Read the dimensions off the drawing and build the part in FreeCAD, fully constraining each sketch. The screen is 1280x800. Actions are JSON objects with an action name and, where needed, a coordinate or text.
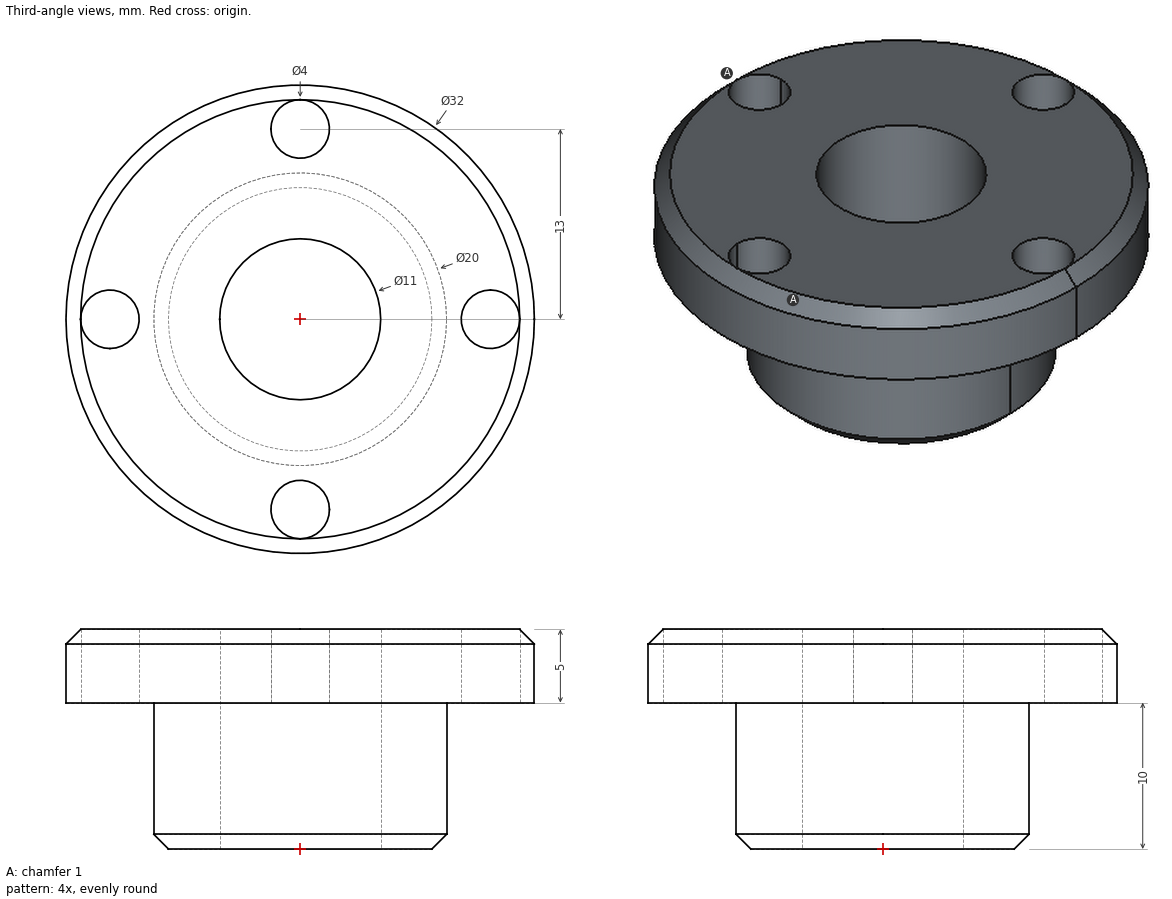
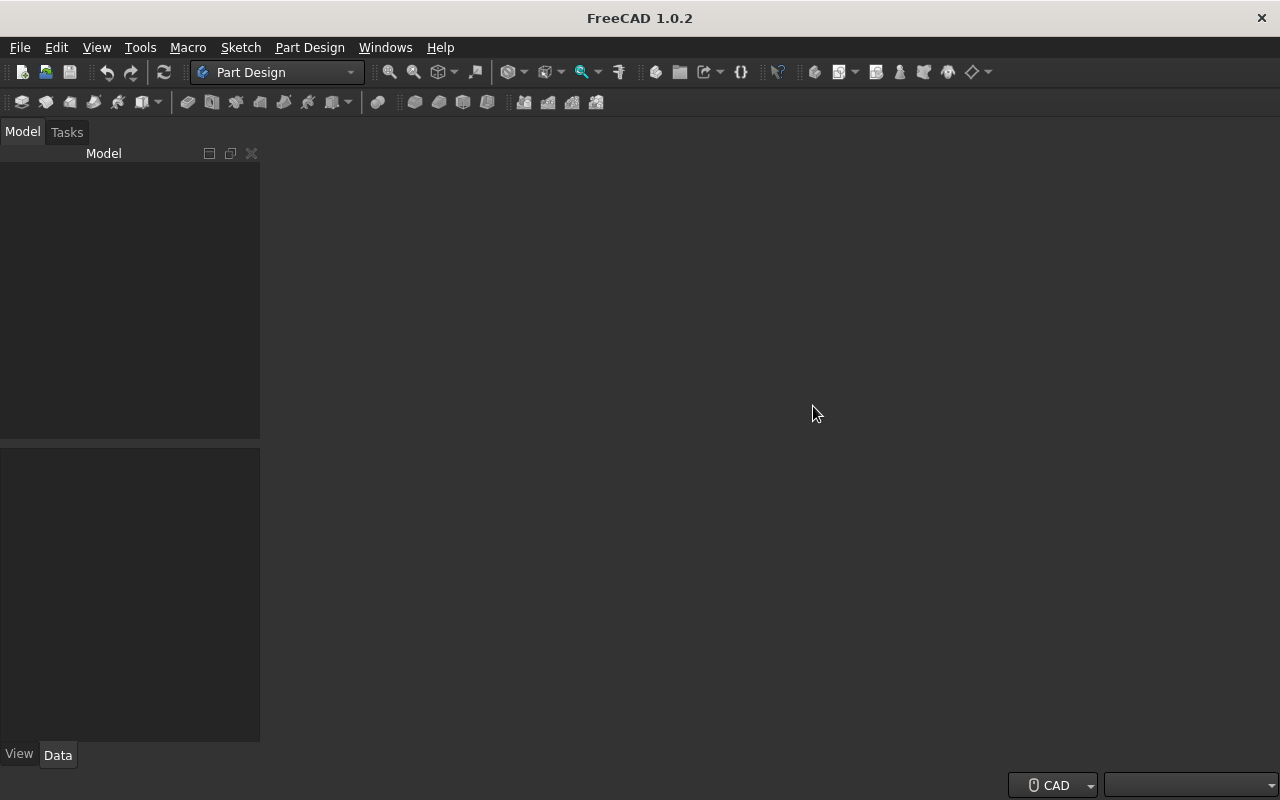
{"action": "left_click", "coordinate": [22, 72]}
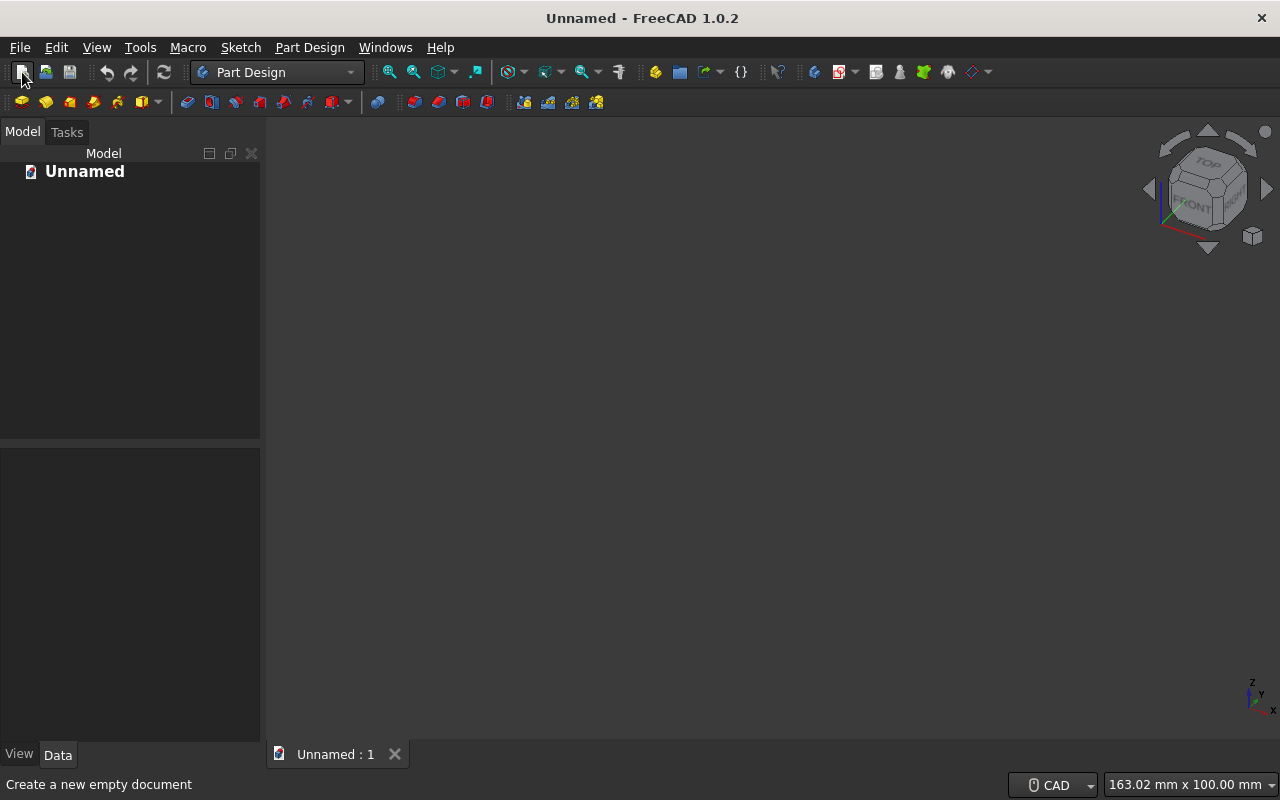
{"action": "left_click", "coordinate": [840, 72]}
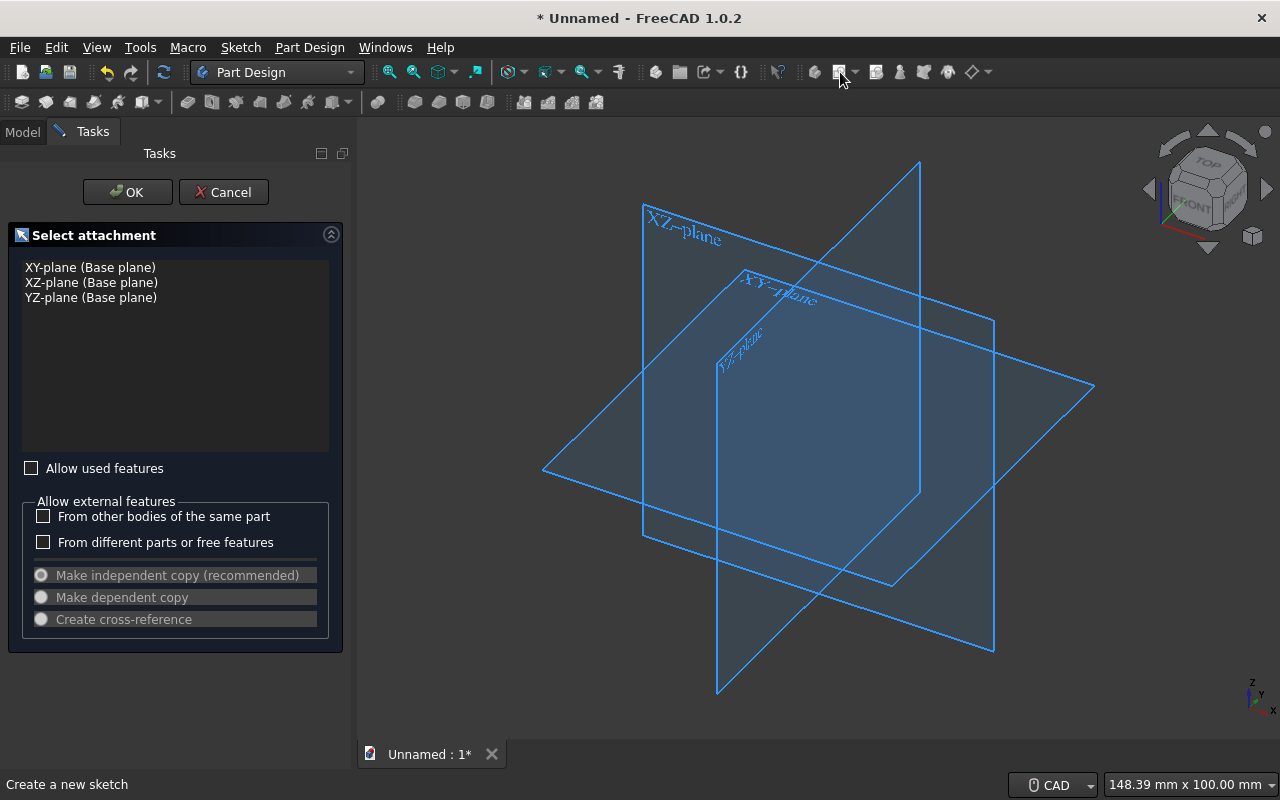
{"action": "left_click", "coordinate": [82, 268]}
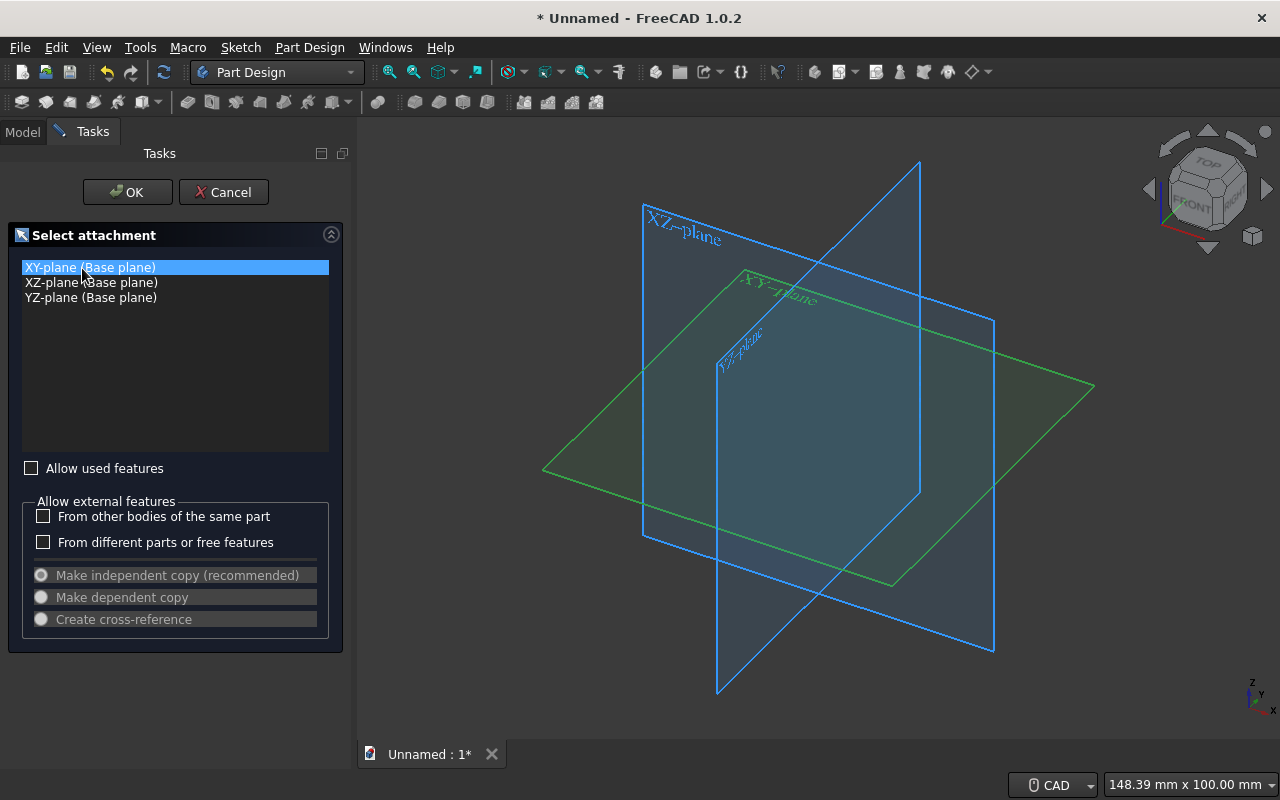
{"action": "left_click", "coordinate": [128, 192]}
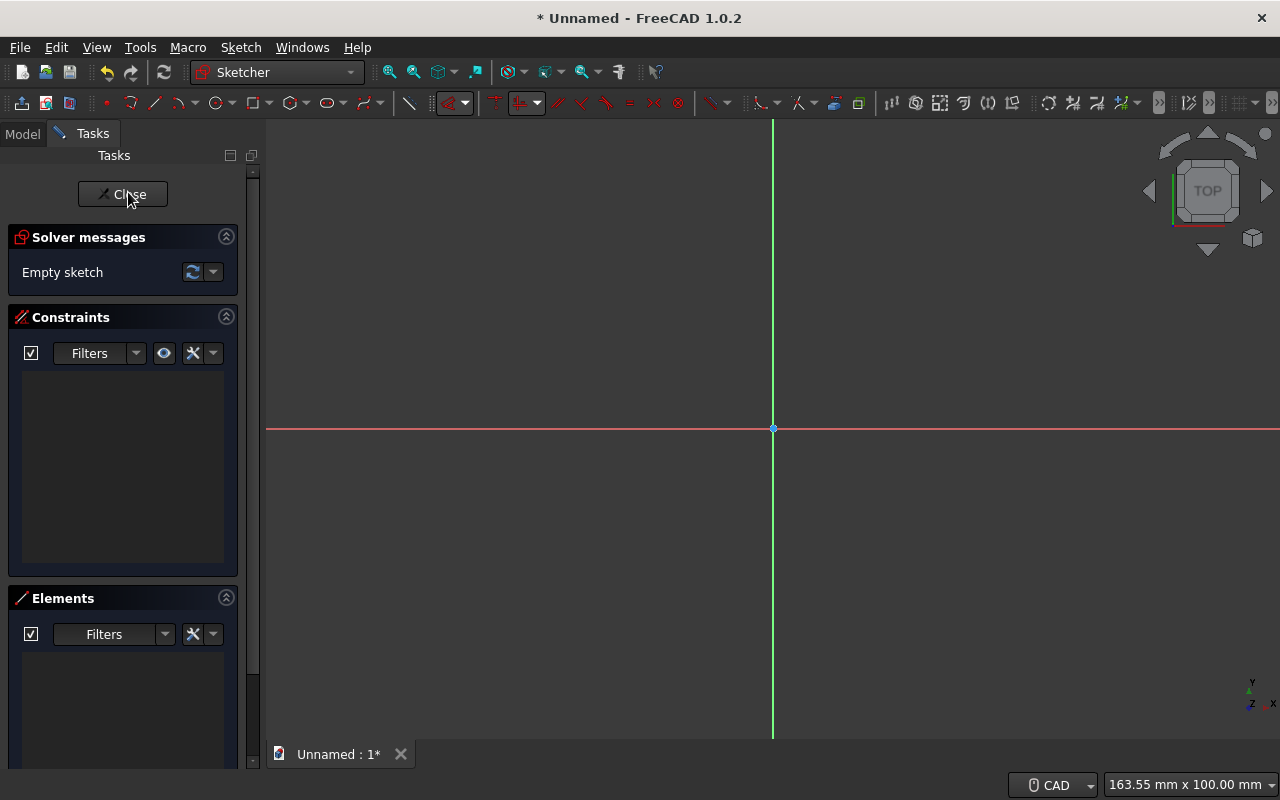
{"action": "scroll", "coordinate": [803, 429], "scroll_direction": "up", "scroll_amount": 6}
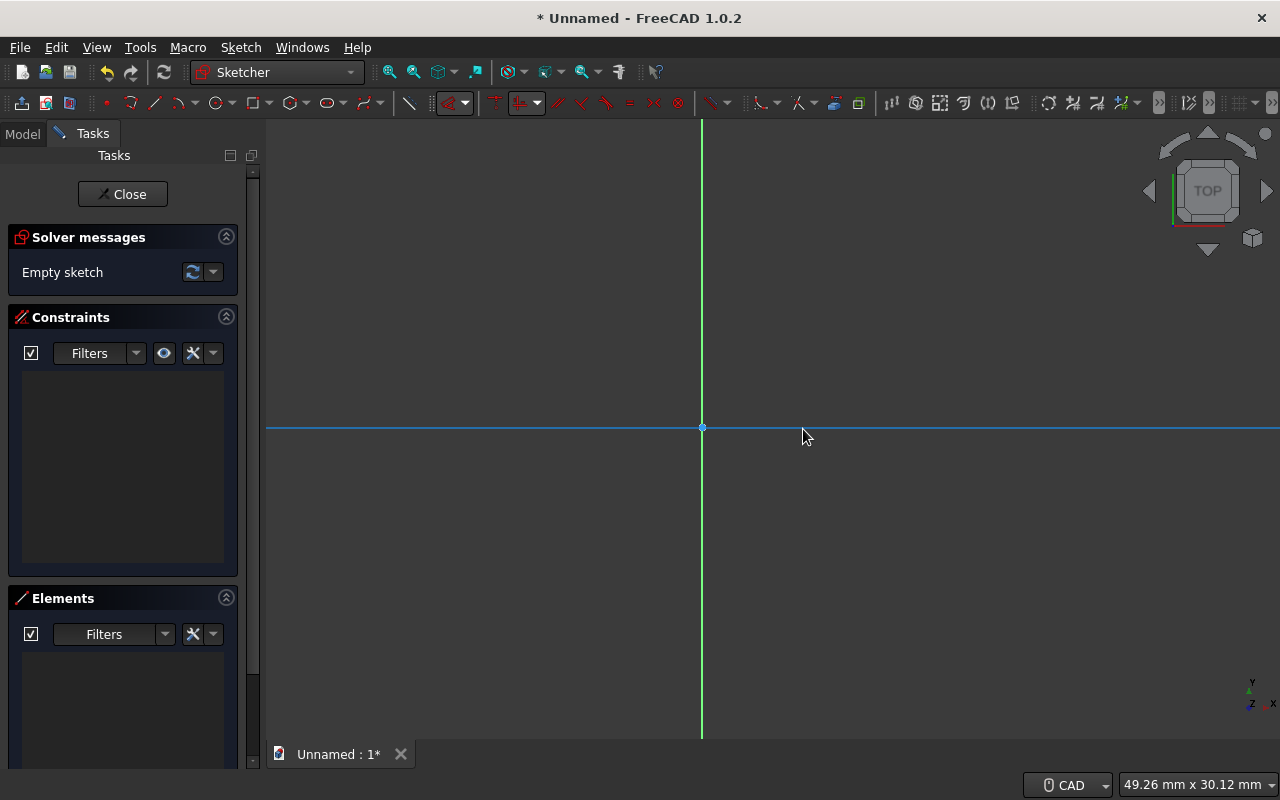
{"action": "left_click", "coordinate": [216, 104]}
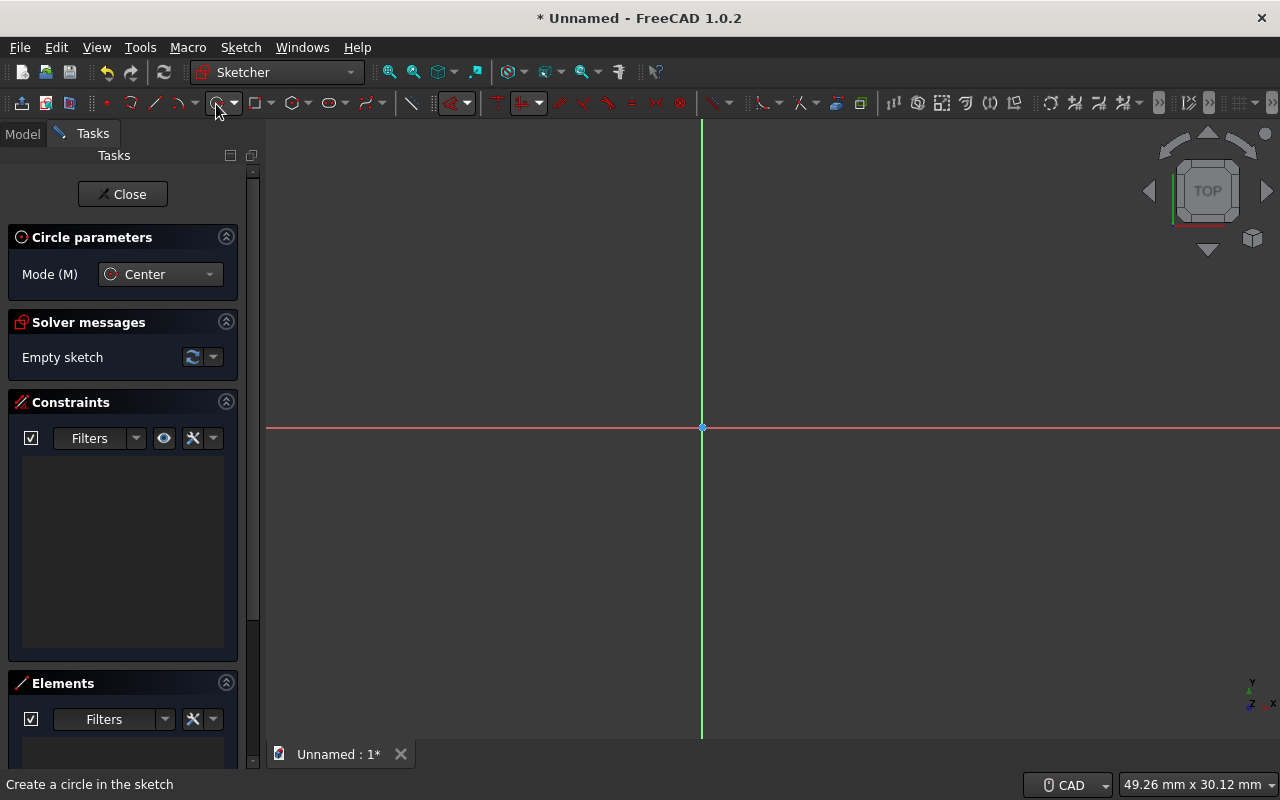
{"action": "left_click", "coordinate": [702, 428]}
{"action": "left_click", "coordinate": [848, 282]}
{"action": "key", "text": "Escape"}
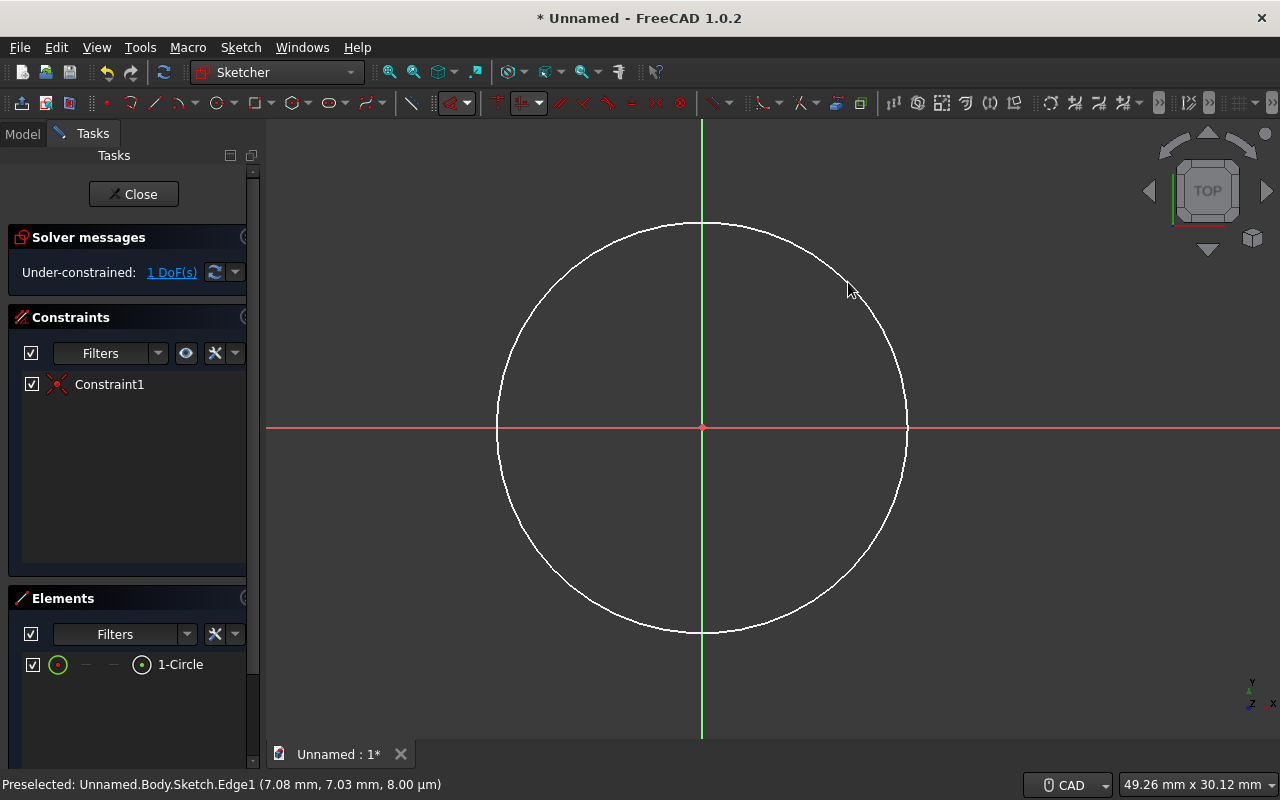
{"action": "left_click", "coordinate": [847, 282]}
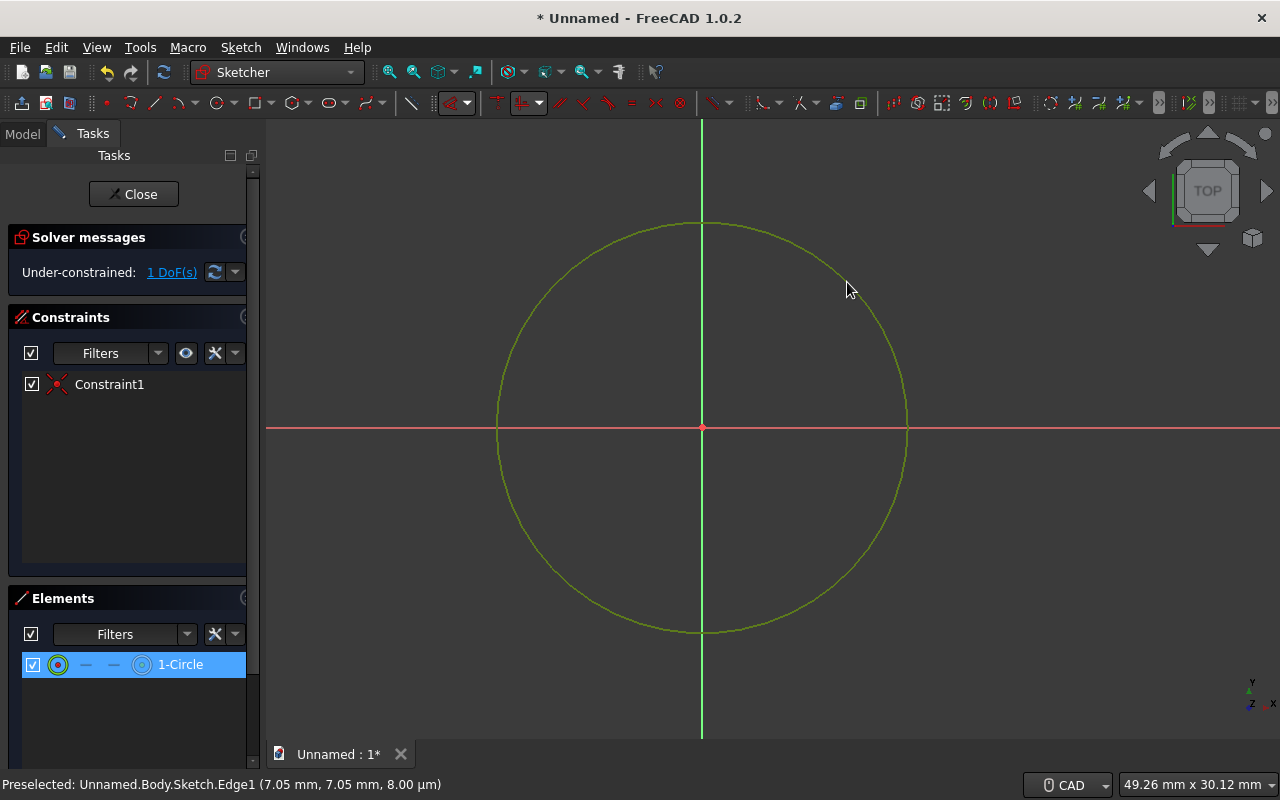
{"action": "key", "text": "k o"}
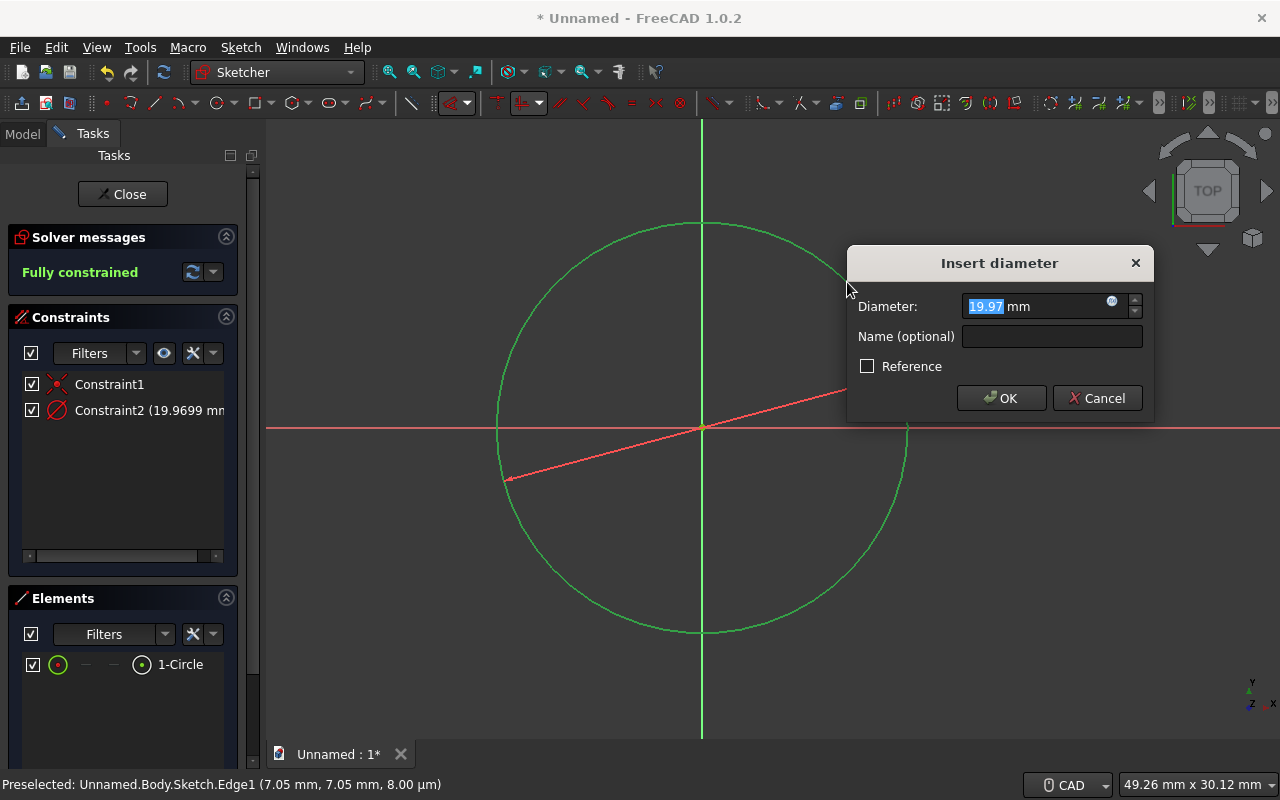
{"action": "type", "text": "20"}
{"action": "key", "text": "Return"}